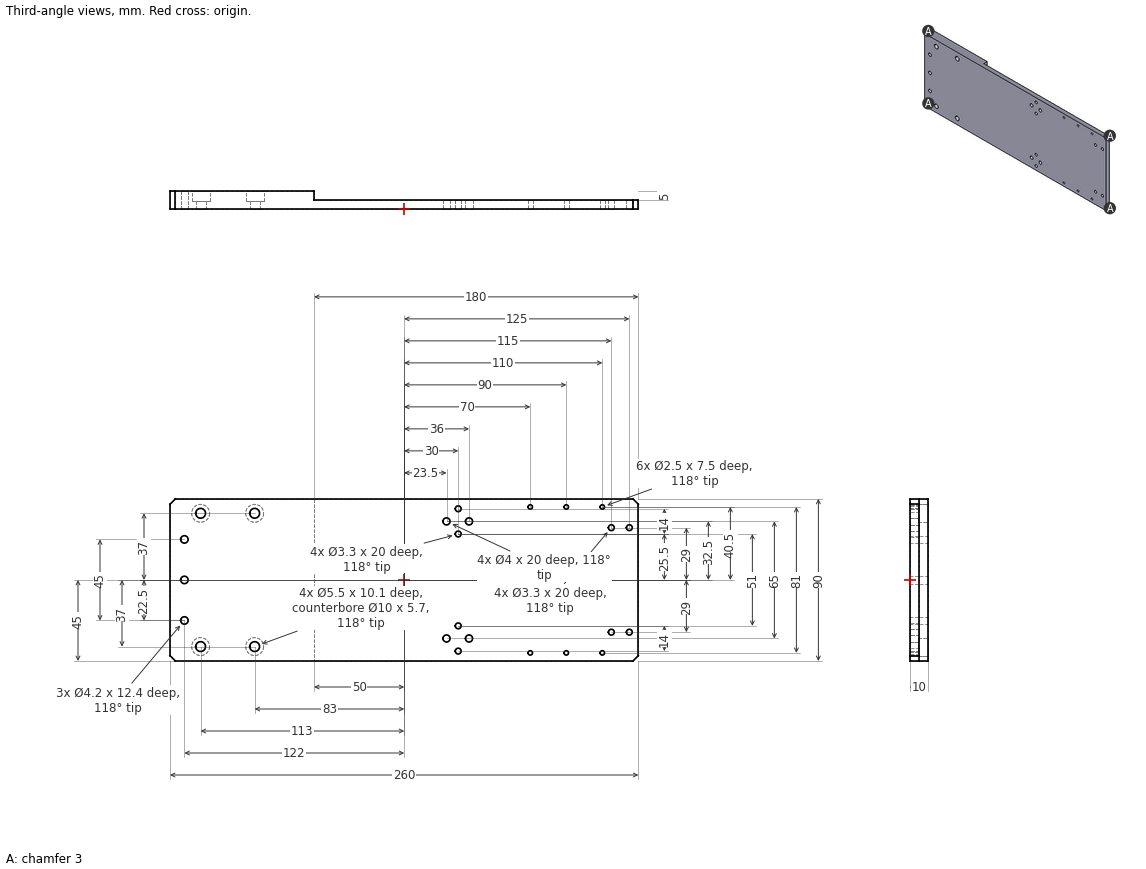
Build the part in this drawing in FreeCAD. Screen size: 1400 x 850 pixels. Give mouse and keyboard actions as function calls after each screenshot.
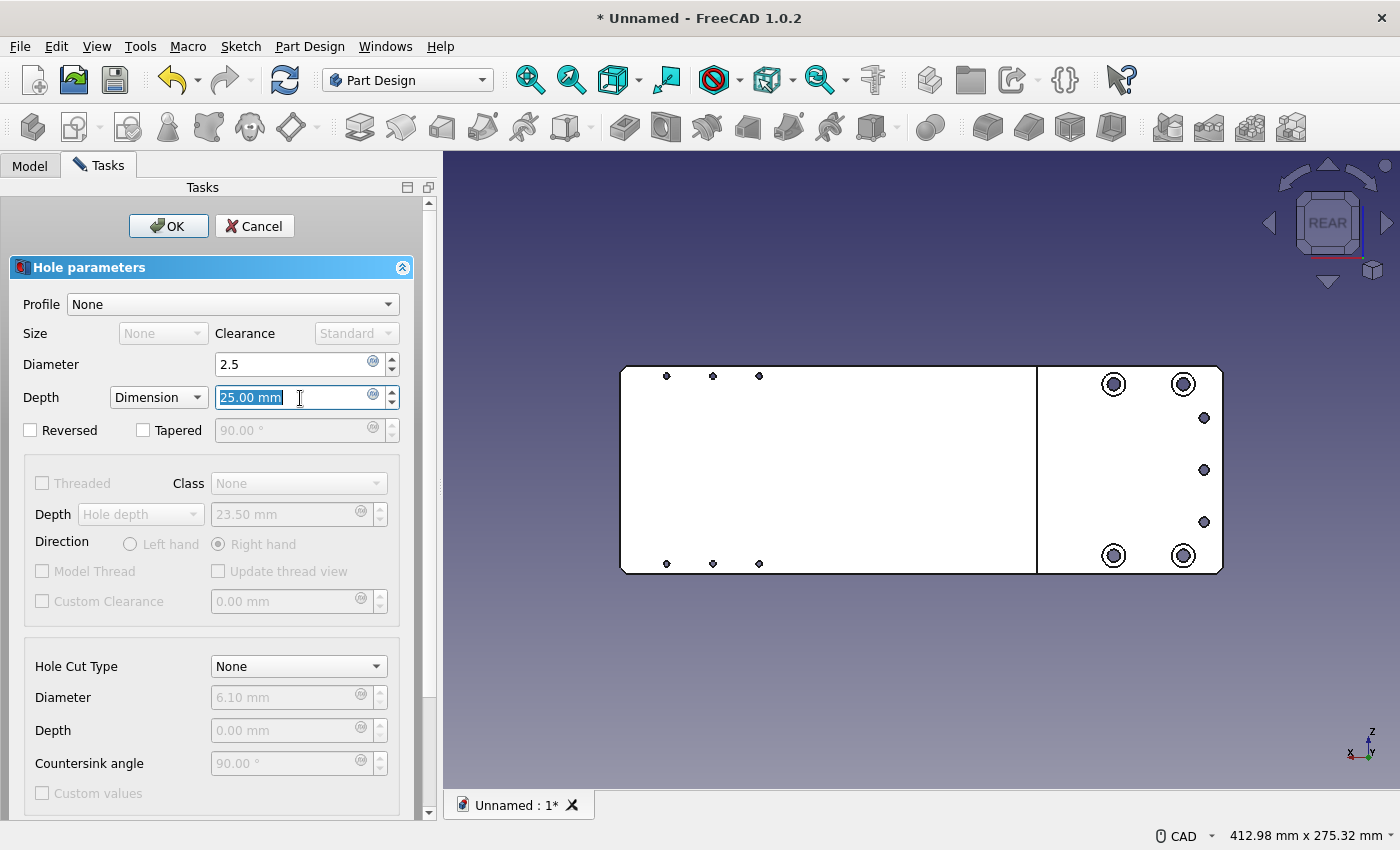
text(7.5)
key(Tab)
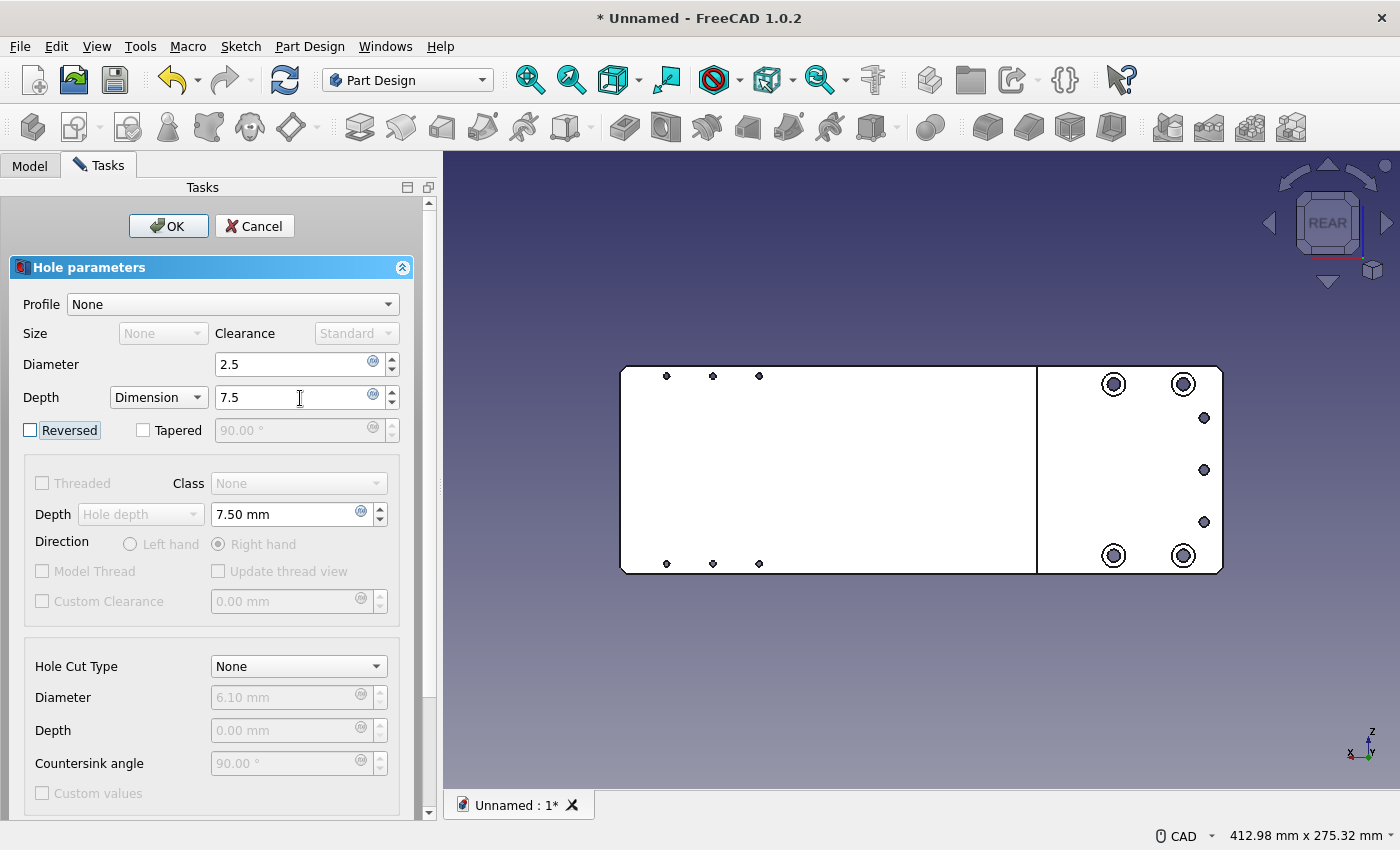
click(169, 226)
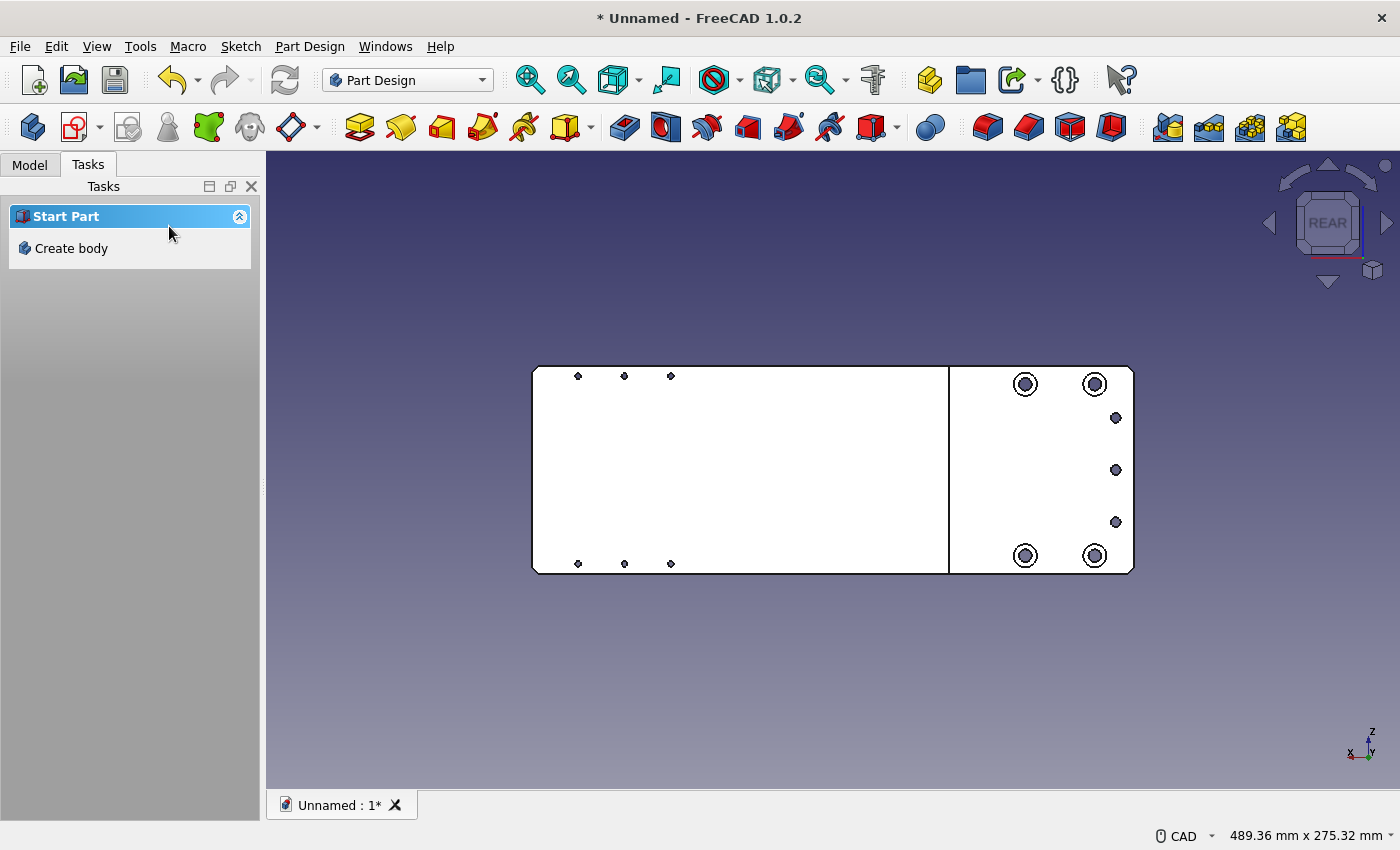
click(740, 469)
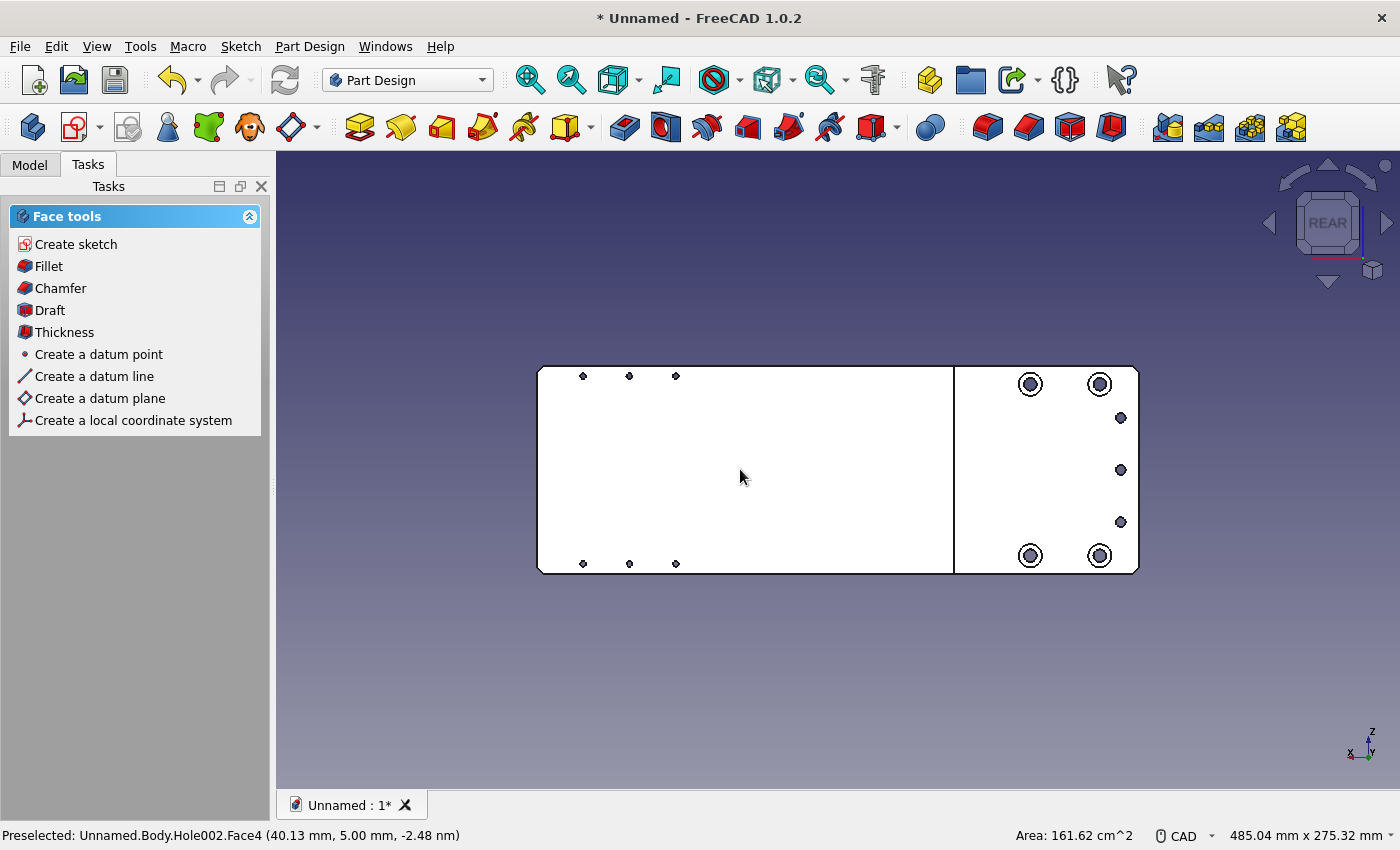
click(74, 128)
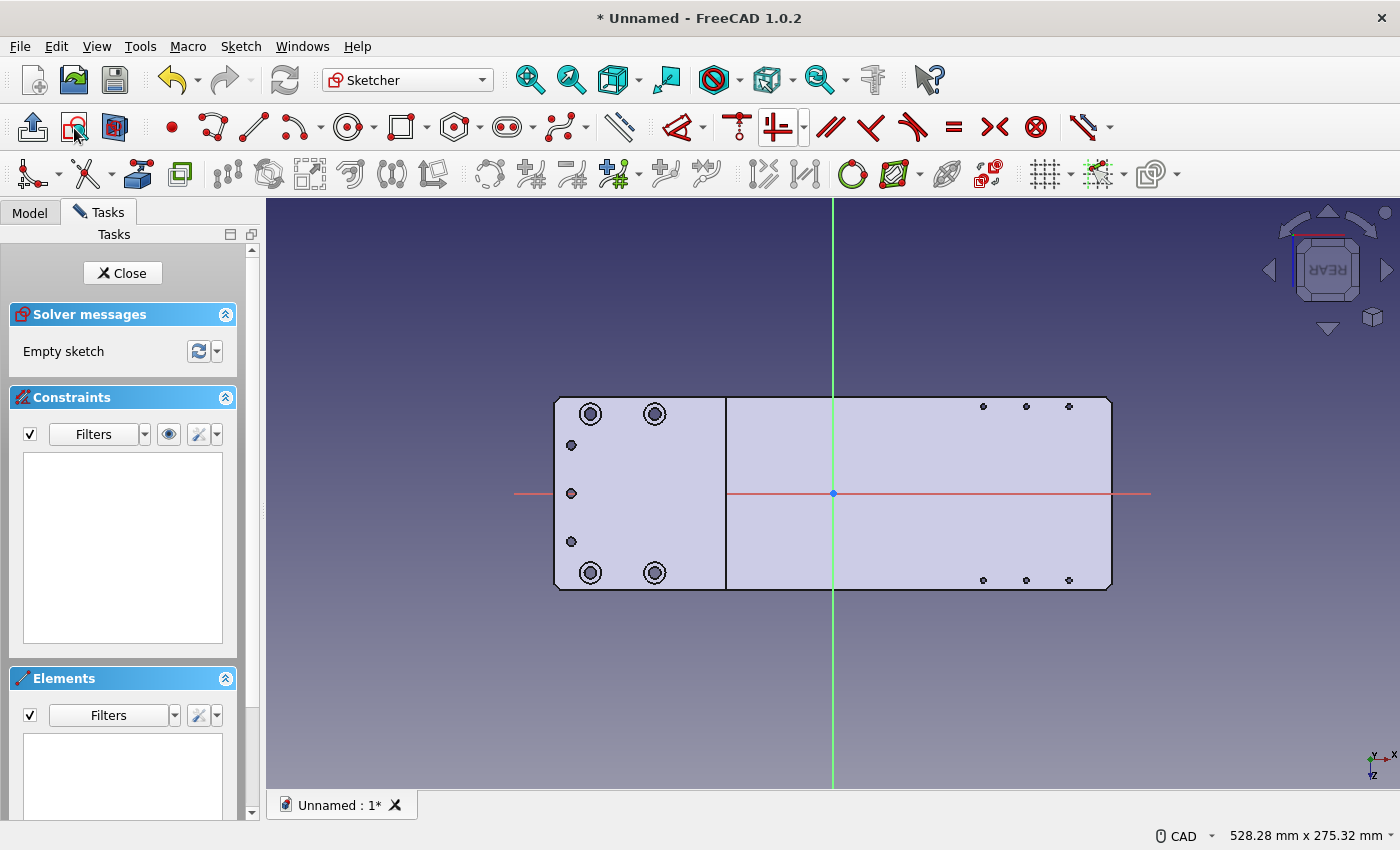
scroll(1136, 493, up, 4)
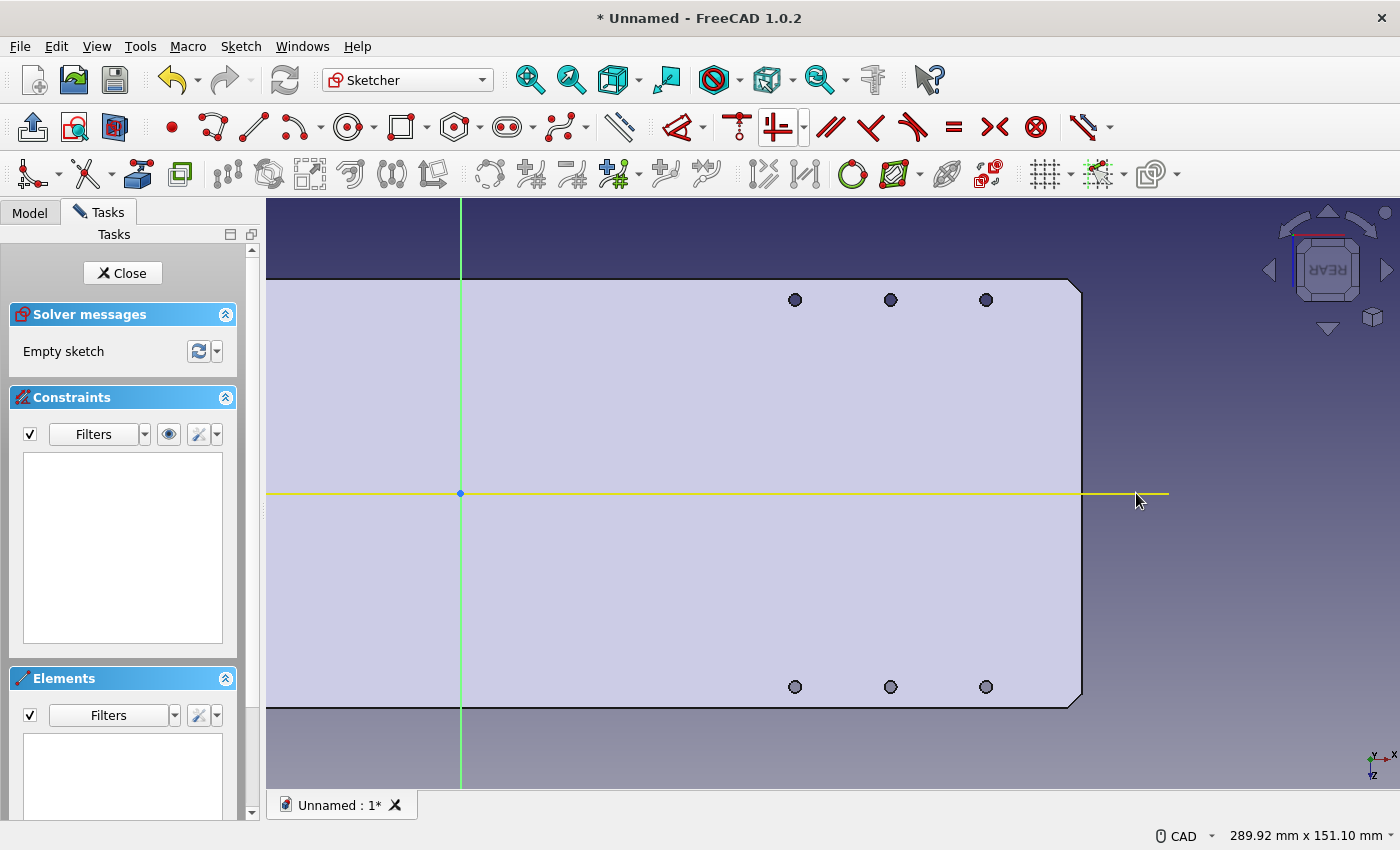
click(348, 128)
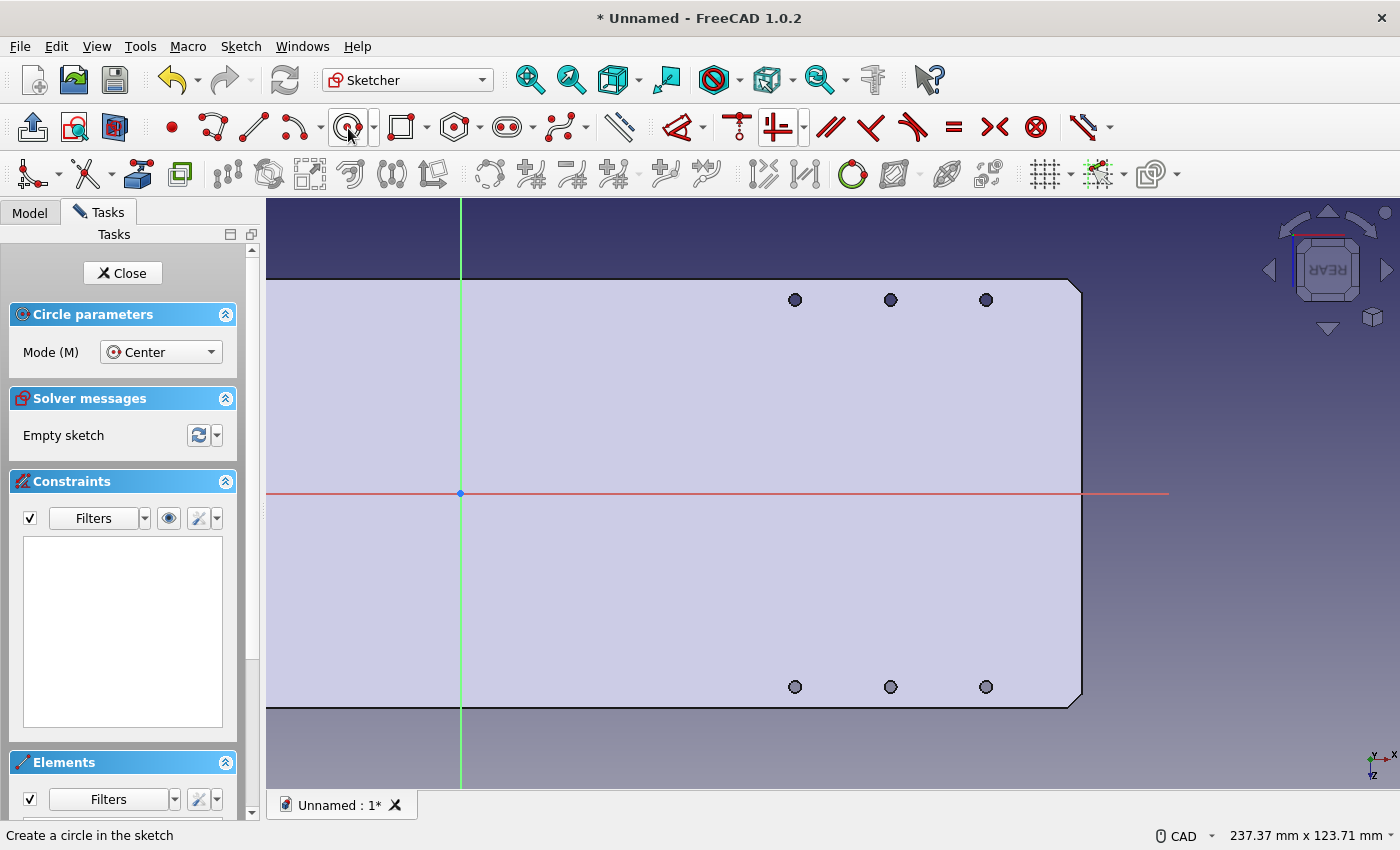
scroll(1010, 632, up, 6)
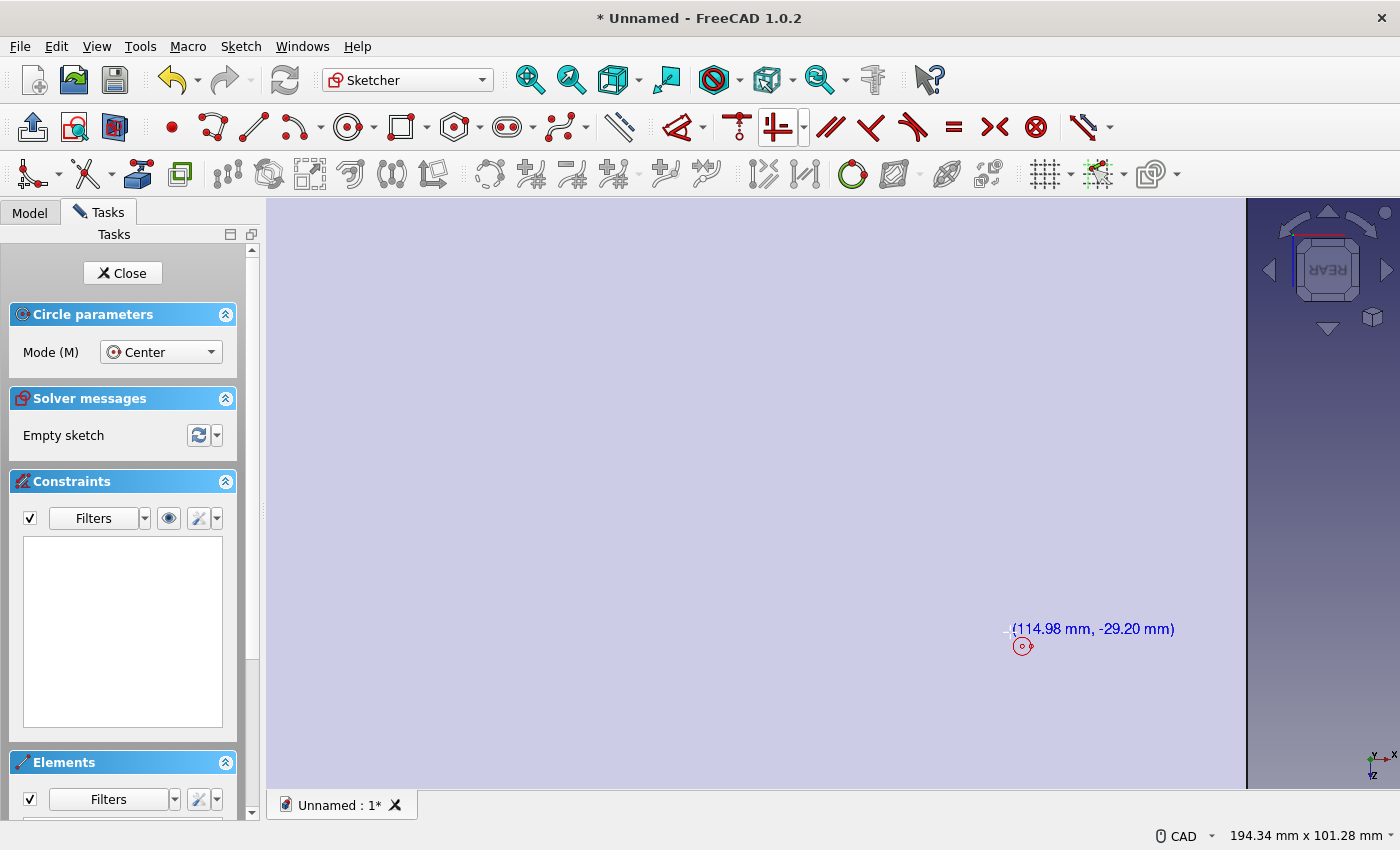
click(1009, 630)
click(1027, 612)